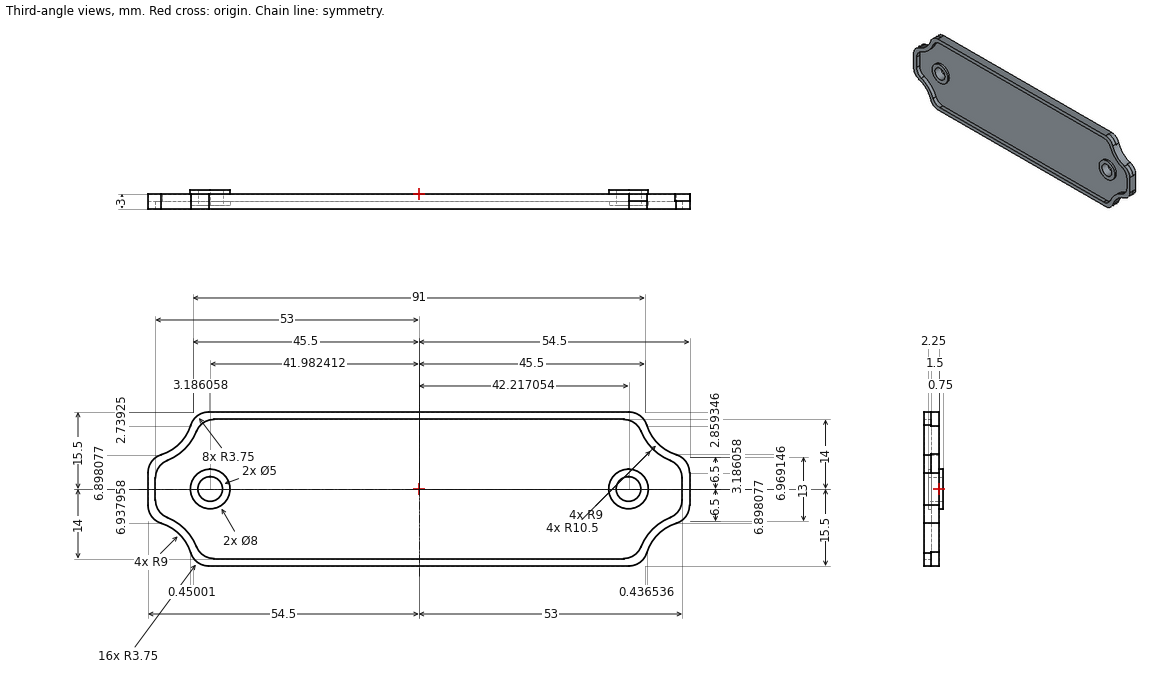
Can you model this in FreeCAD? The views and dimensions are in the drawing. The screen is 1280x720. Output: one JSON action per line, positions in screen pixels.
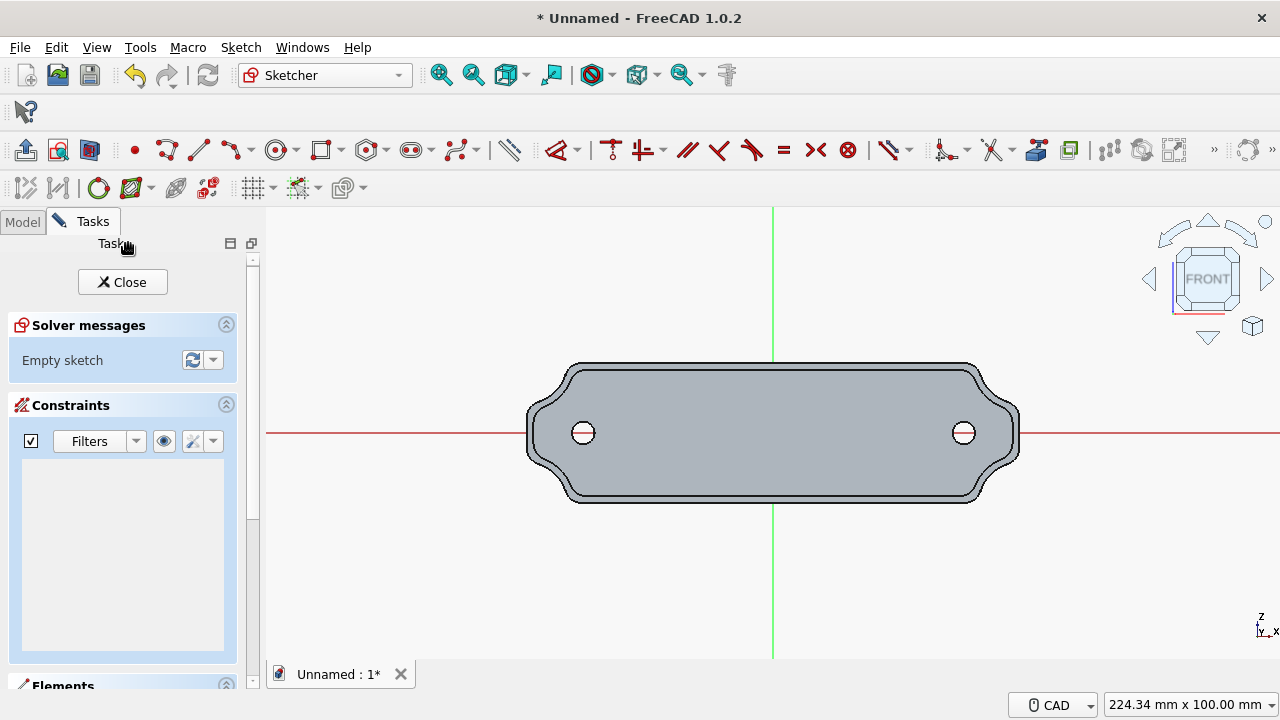
{"action": "left_click", "coordinate": [90, 150]}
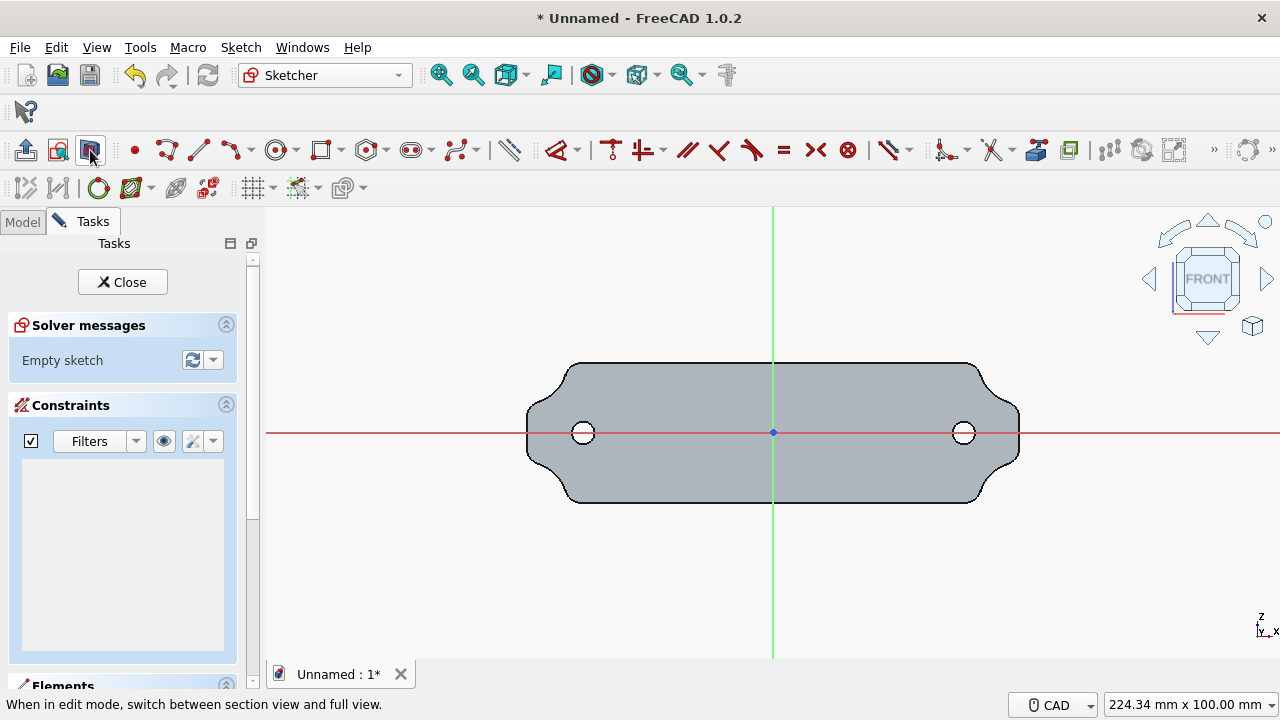
{"action": "scroll", "coordinate": [914, 433], "scroll_direction": "up", "scroll_amount": 2}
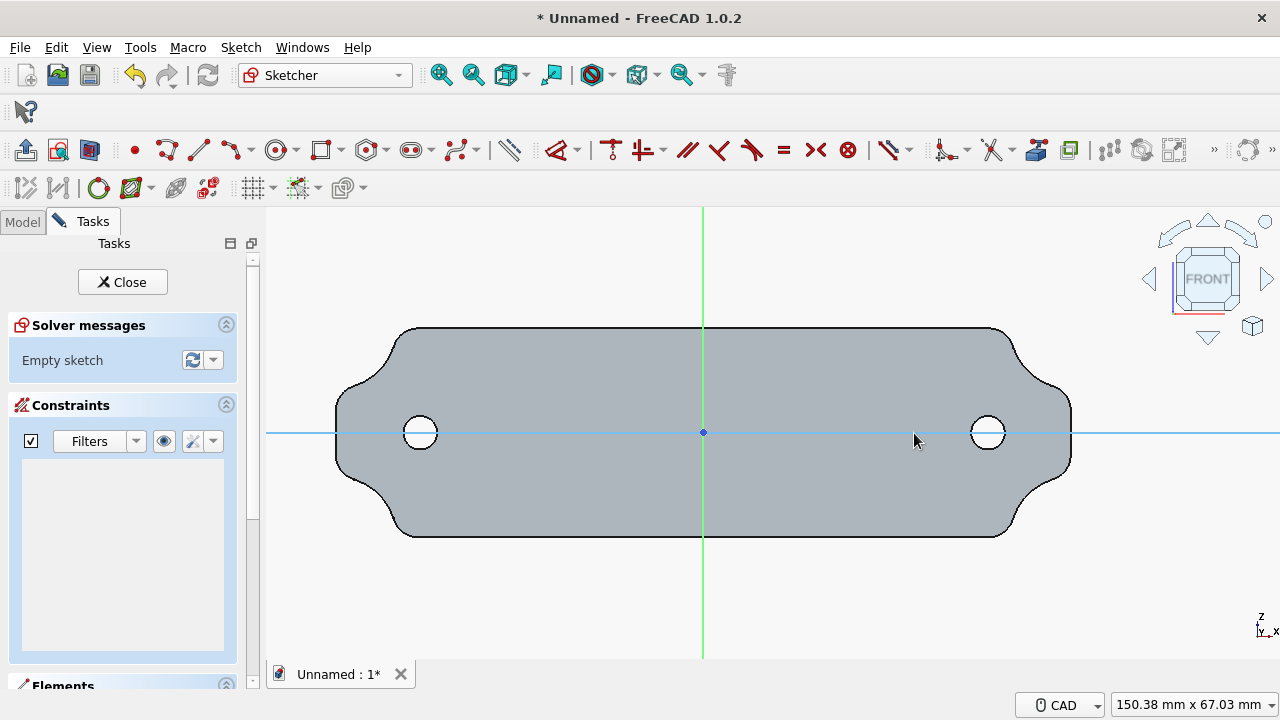
{"action": "left_click", "coordinate": [276, 150]}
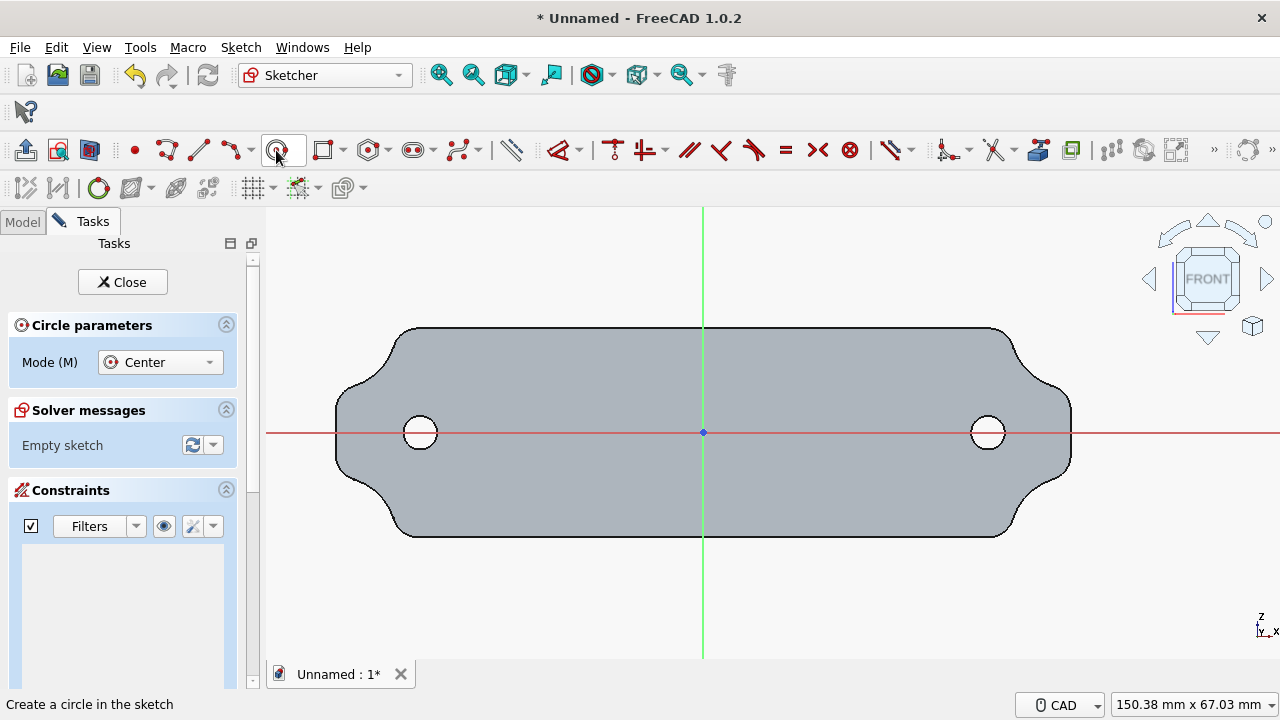
{"action": "left_click", "coordinate": [420, 433]}
{"action": "mouse_move", "coordinate": [439, 414]}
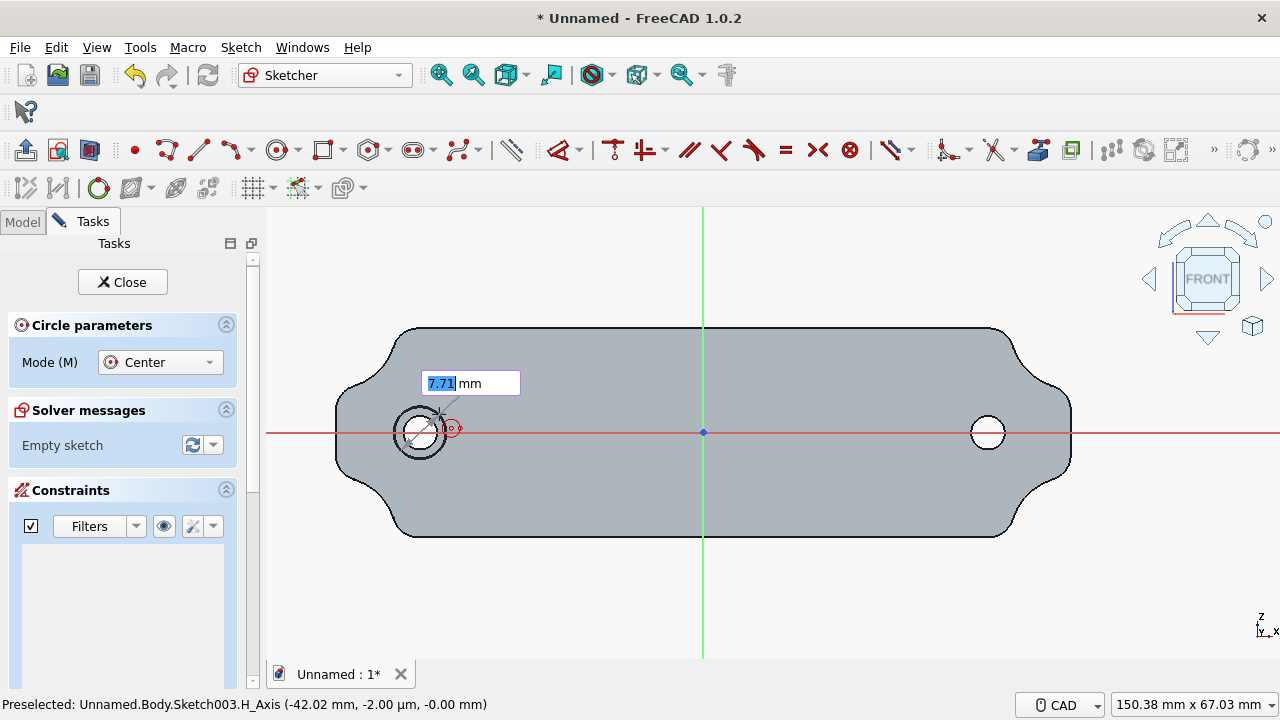
{"action": "type", "text": "8"}
{"action": "key", "text": "Return"}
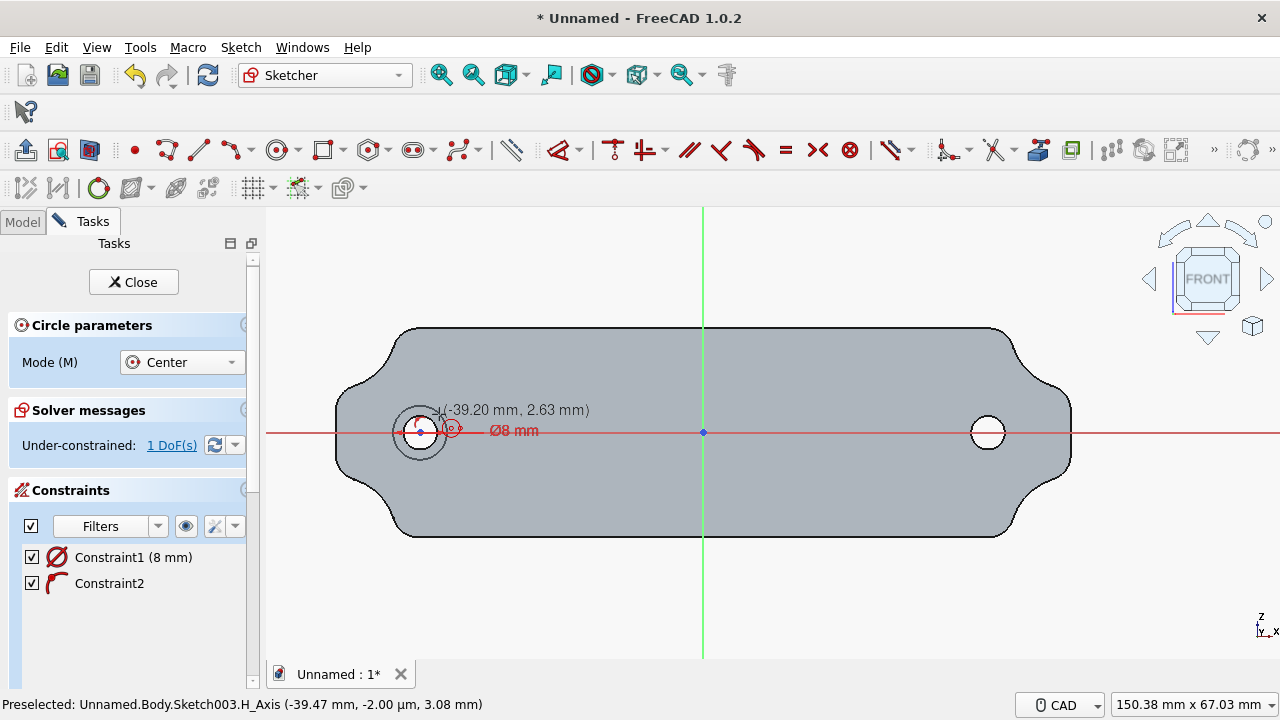
{"action": "left_click", "coordinate": [988, 433]}
{"action": "mouse_move", "coordinate": [1007, 414]}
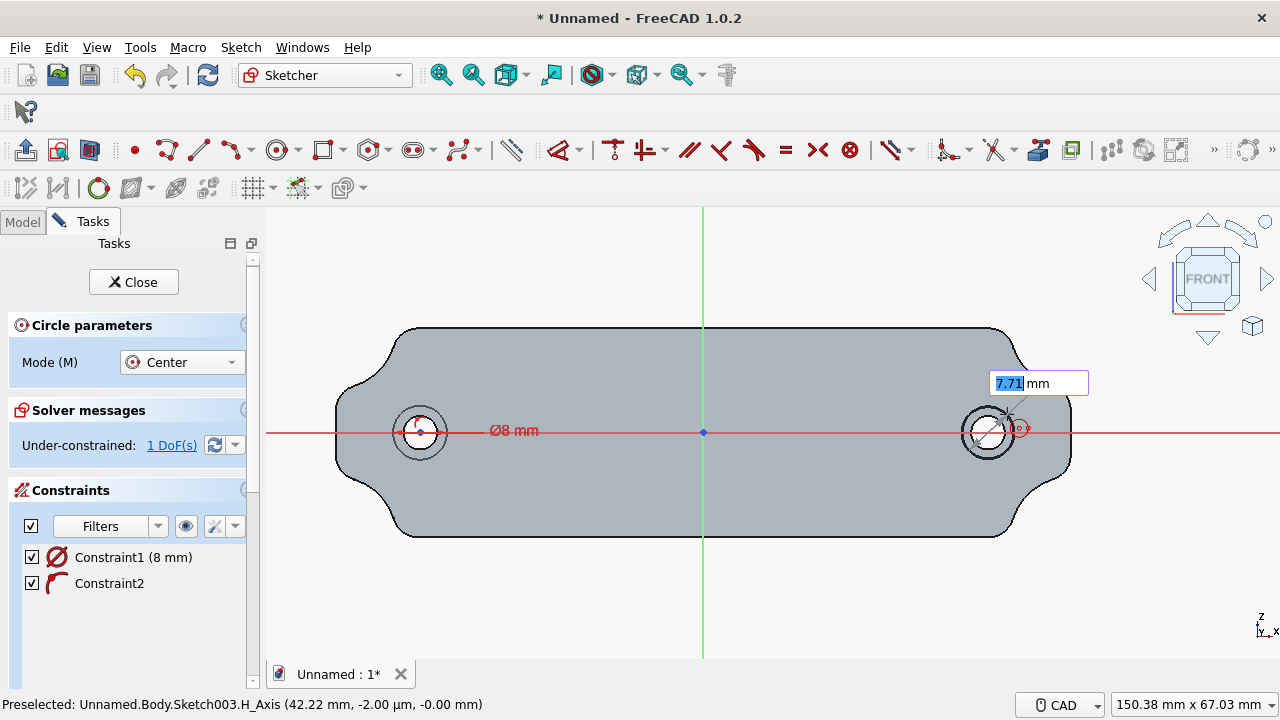
{"action": "type", "text": "8"}
{"action": "key", "text": "Return"}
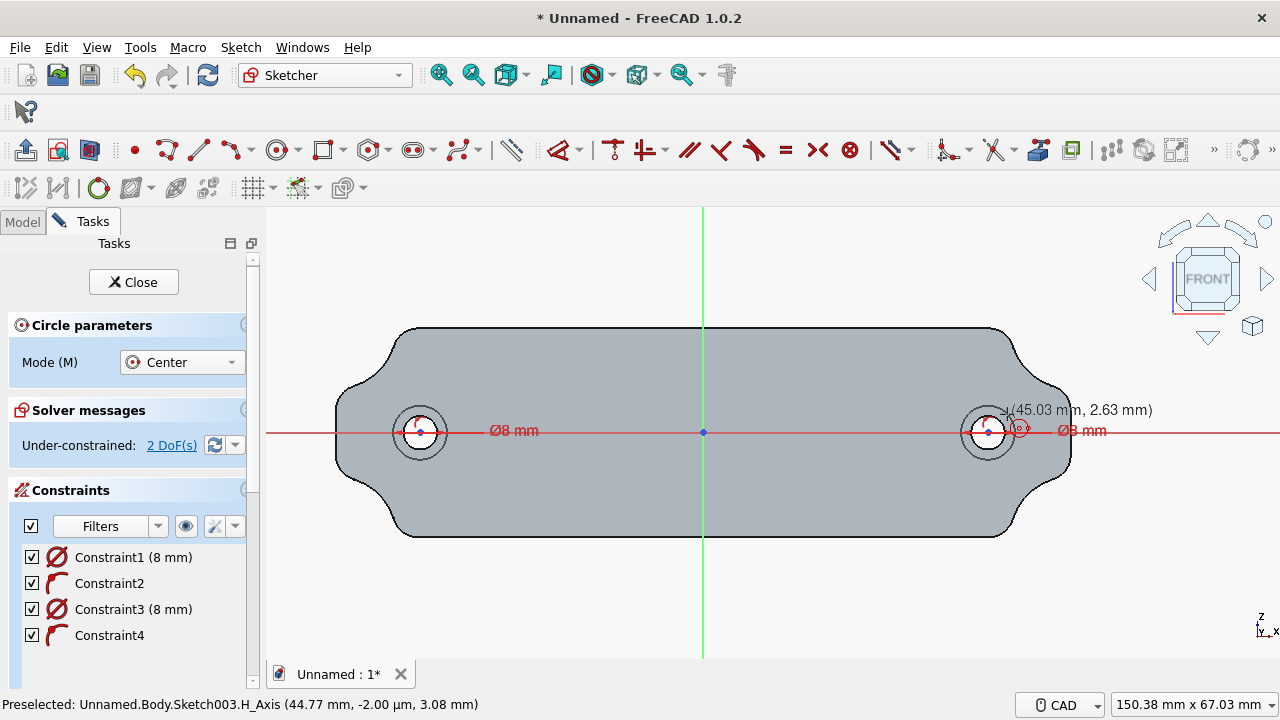
{"action": "scroll", "coordinate": [420, 433], "scroll_direction": "up", "scroll_amount": 2}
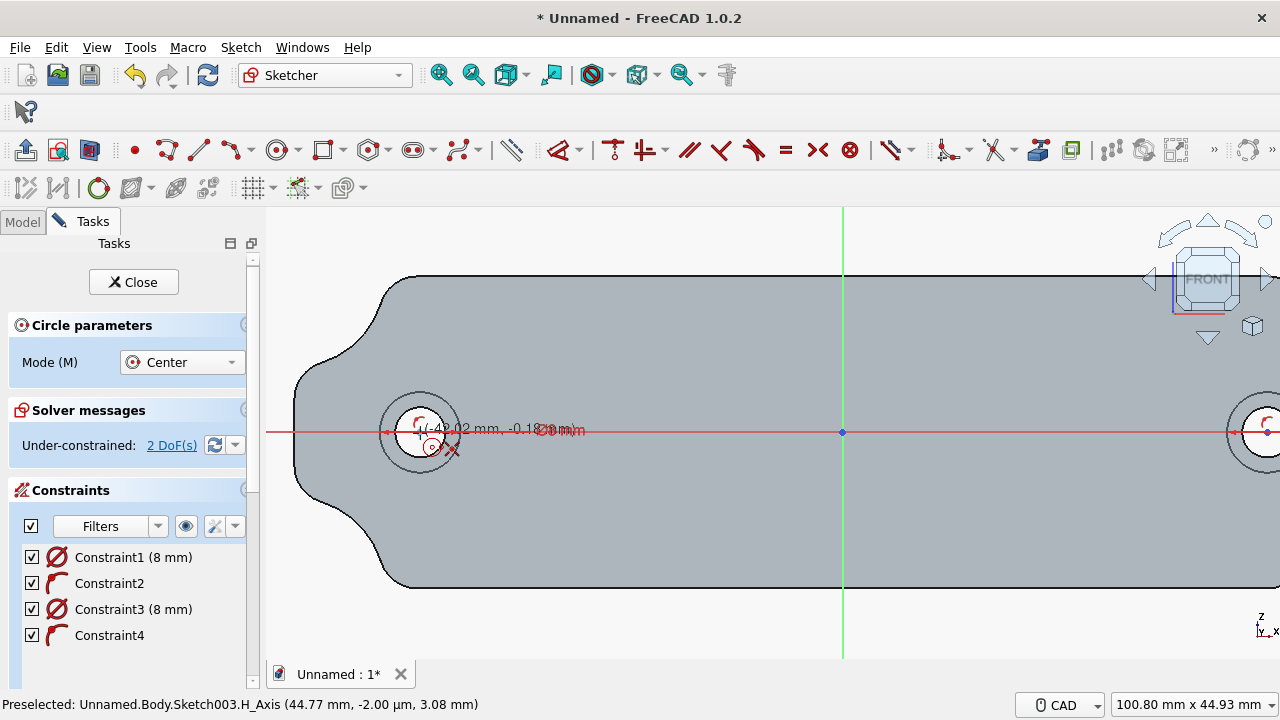
{"action": "left_click", "coordinate": [420, 432]}
{"action": "mouse_move", "coordinate": [438, 415]}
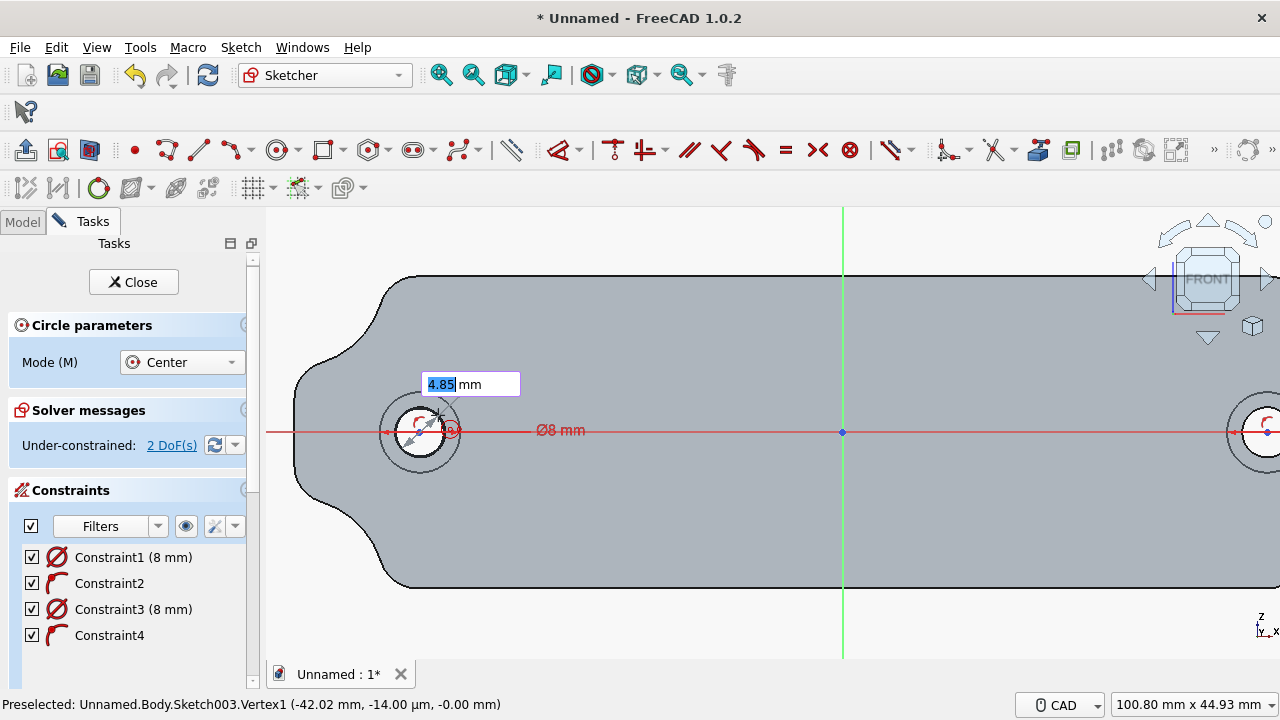
{"action": "type", "text": "5"}
{"action": "key", "text": "Return"}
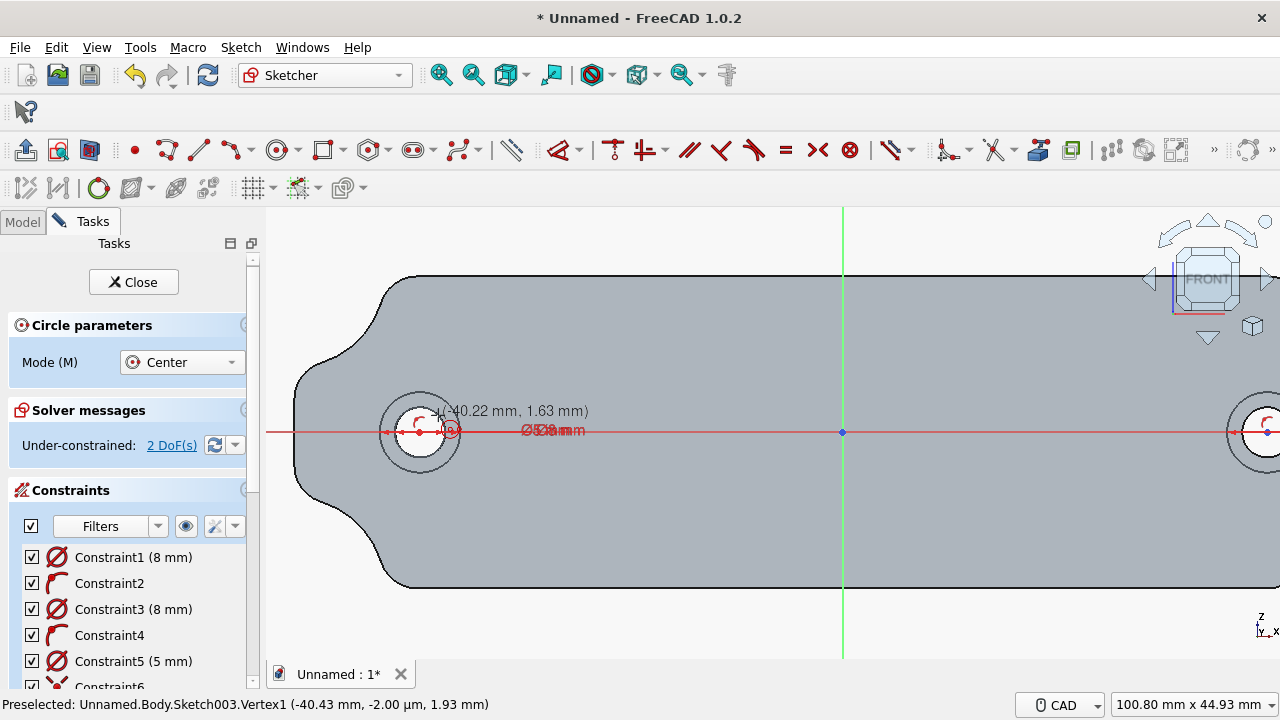
{"action": "scroll", "coordinate": [421, 434], "scroll_direction": "down", "scroll_amount": 2}